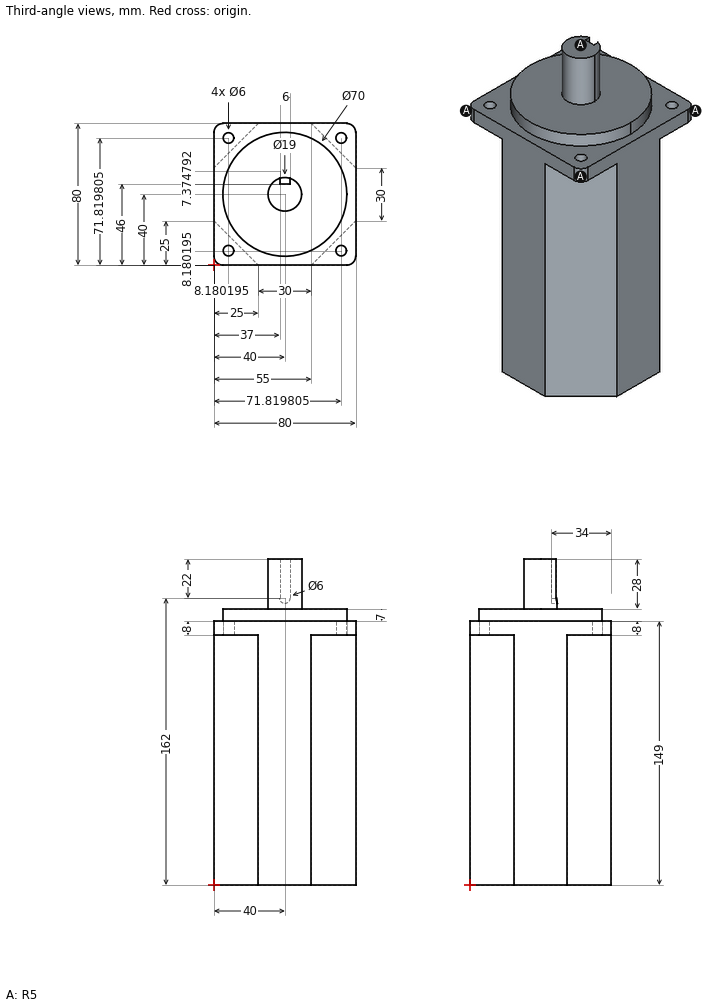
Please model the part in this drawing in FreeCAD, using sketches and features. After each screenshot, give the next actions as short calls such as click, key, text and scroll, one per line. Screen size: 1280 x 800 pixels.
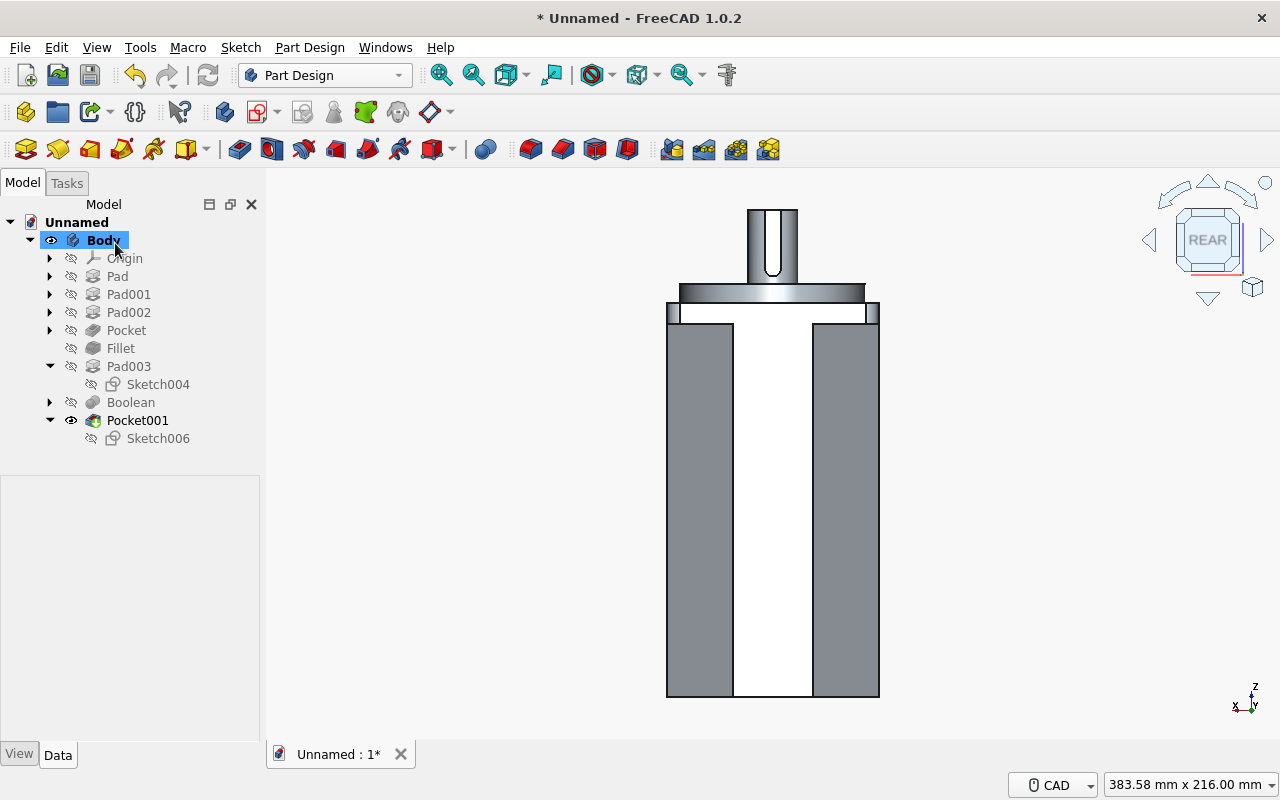
key(0)